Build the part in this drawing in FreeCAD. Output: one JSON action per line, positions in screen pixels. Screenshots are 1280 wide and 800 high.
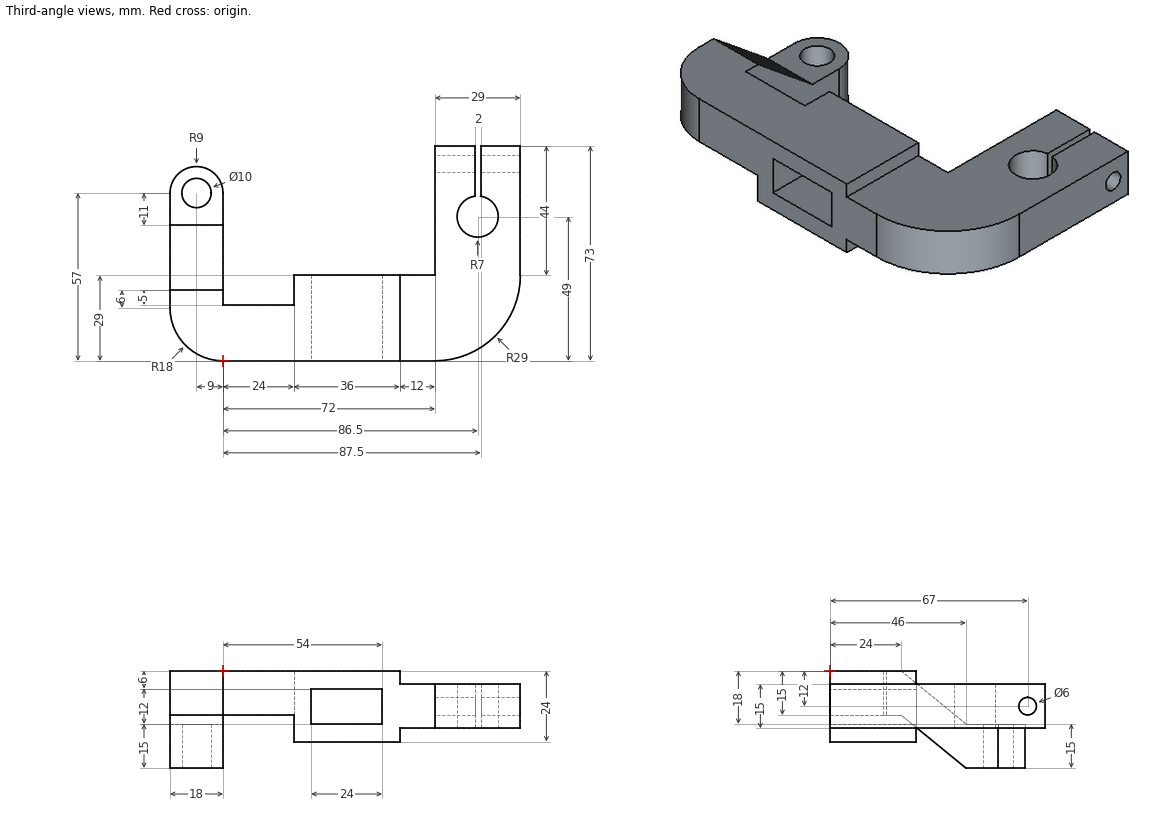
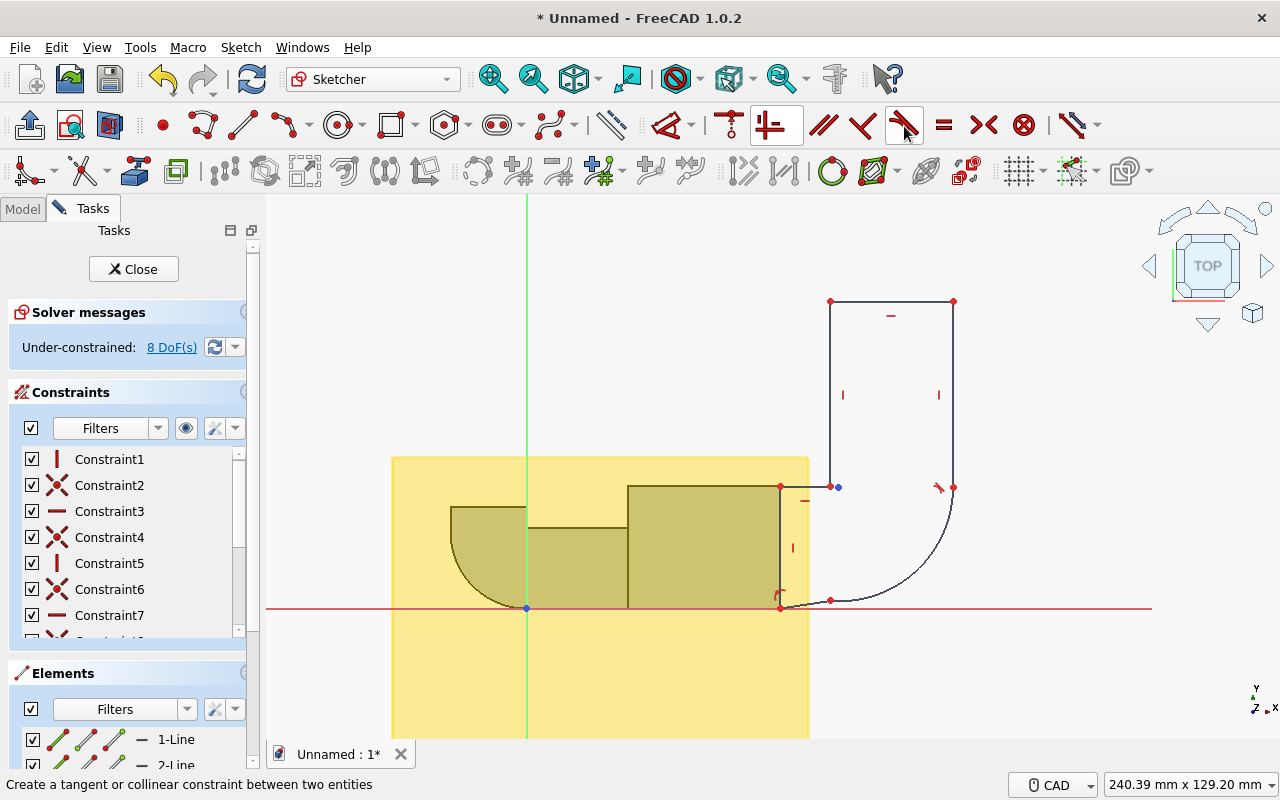
{"action": "left_click", "coordinate": [795, 606]}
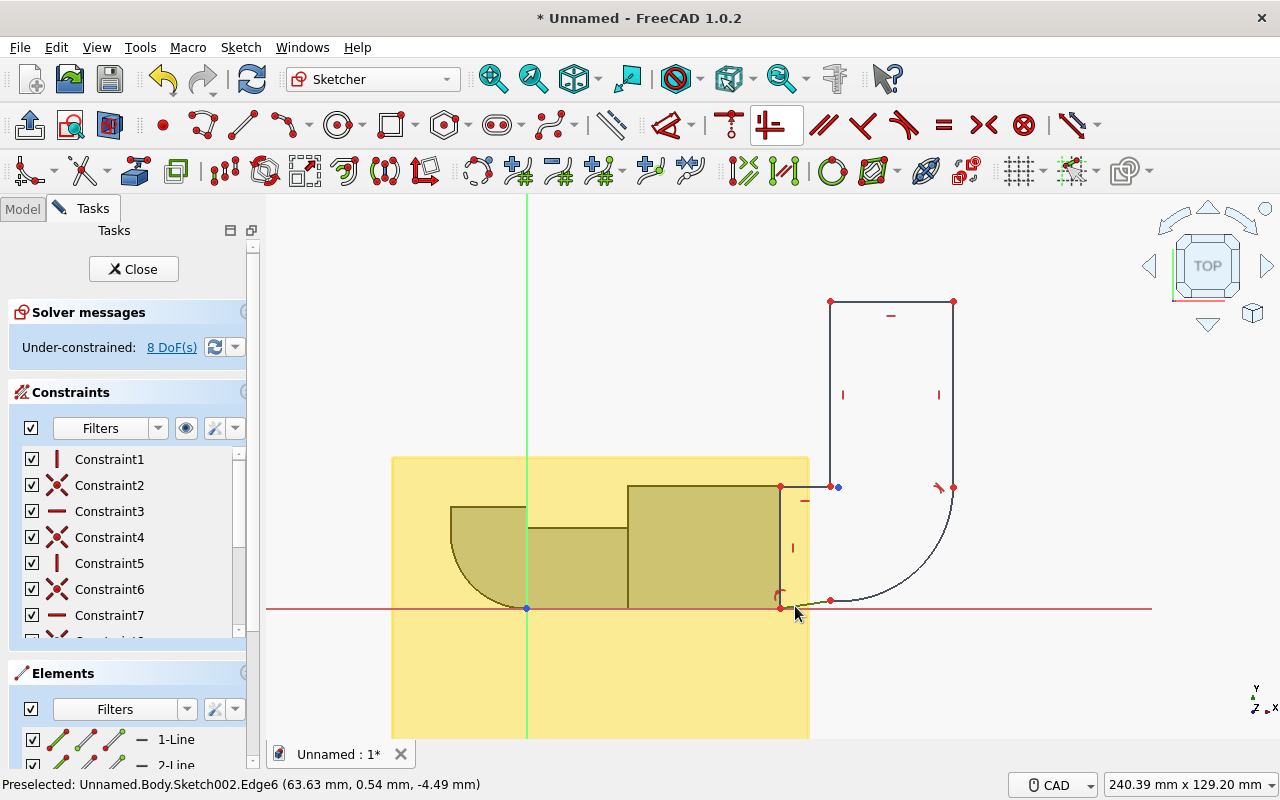
{"action": "left_click", "coordinate": [885, 591]}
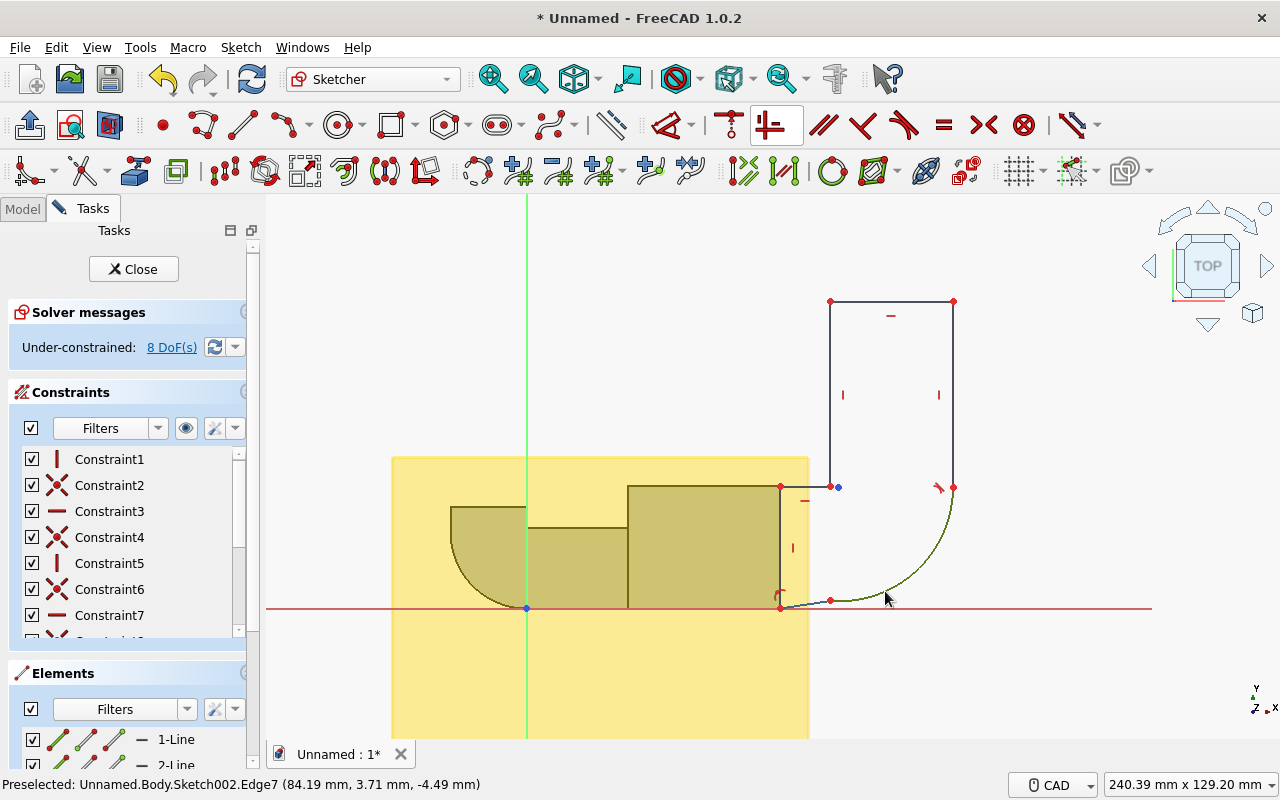
{"action": "left_click", "coordinate": [904, 126]}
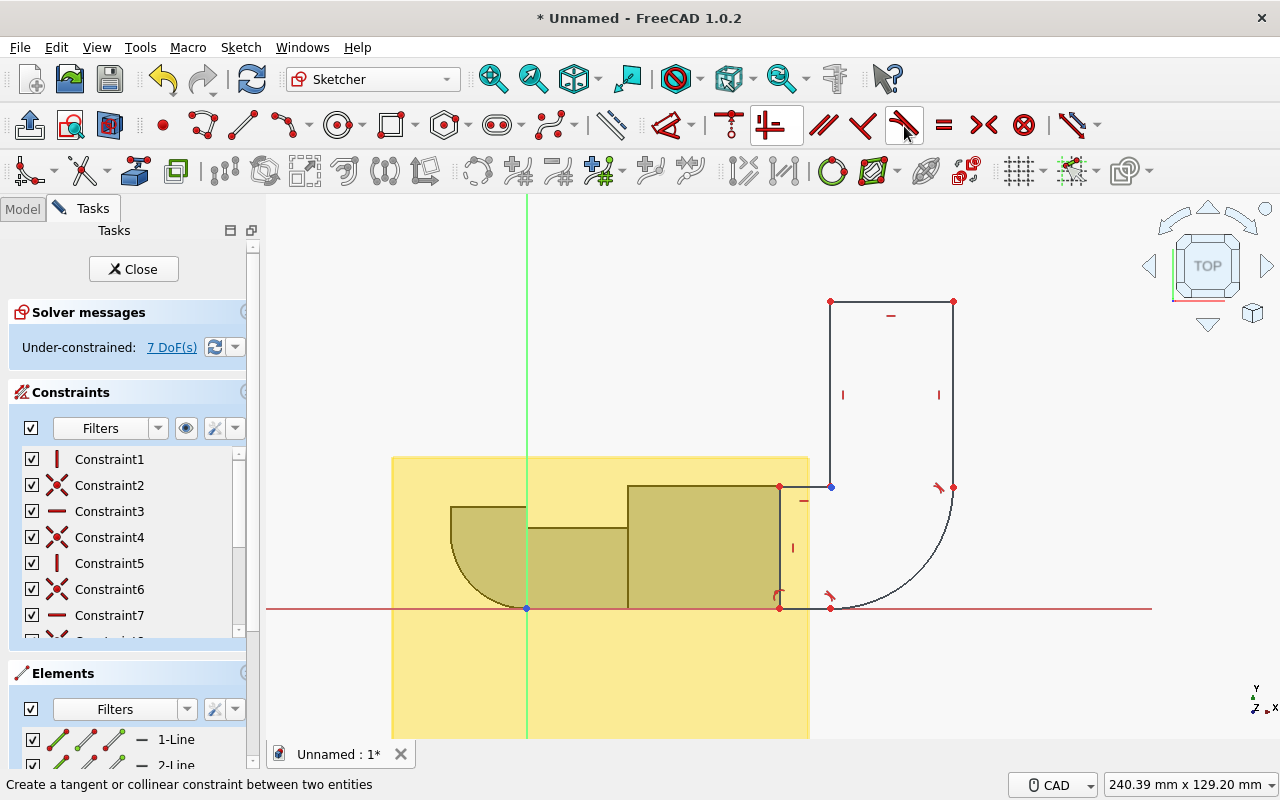
{"action": "left_click", "coordinate": [795, 609]}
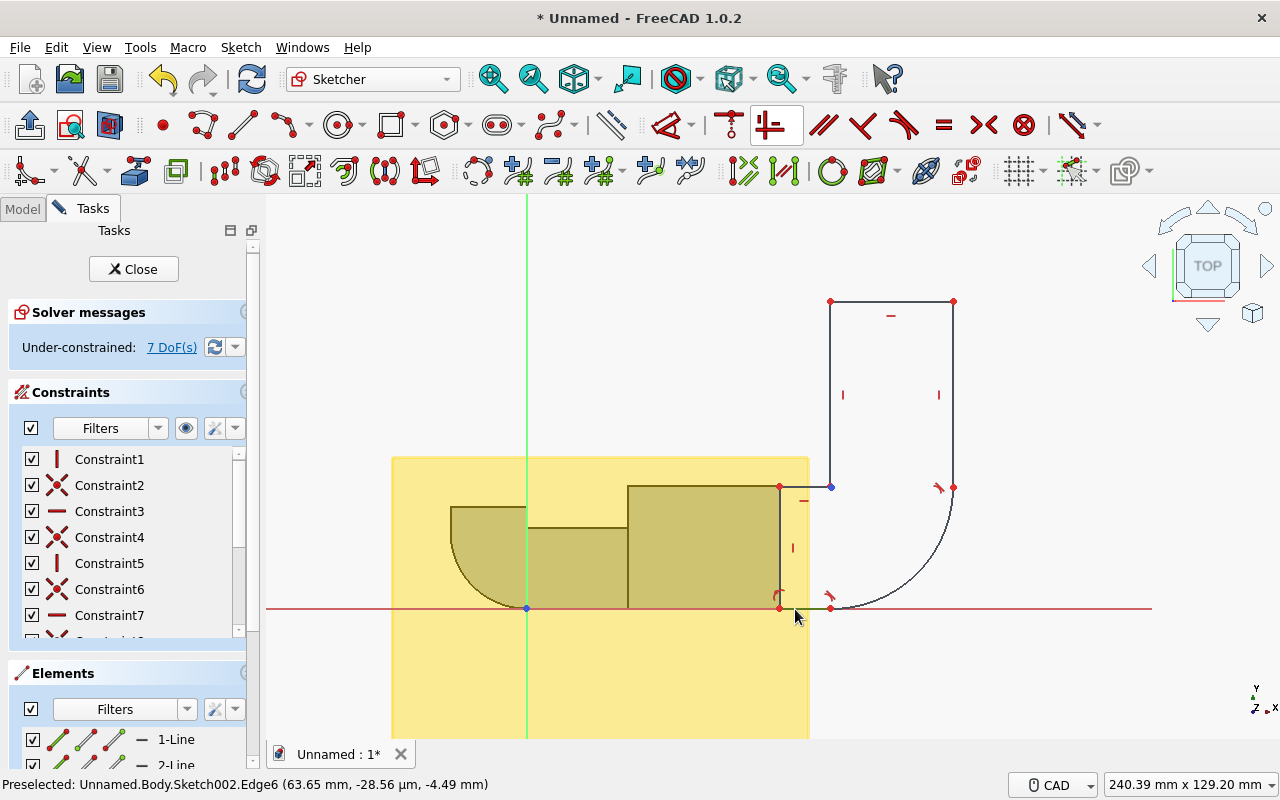
{"action": "left_click", "coordinate": [798, 126]}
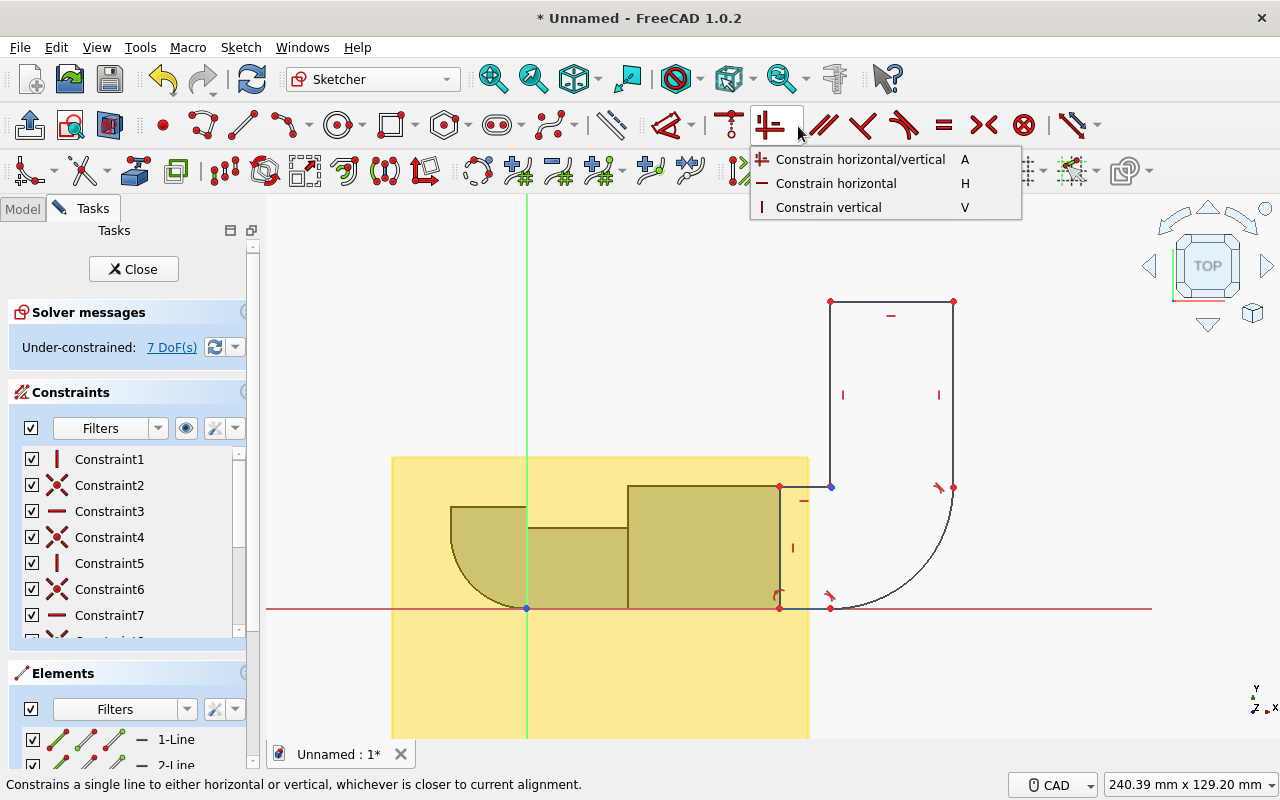
{"action": "left_click", "coordinate": [886, 183]}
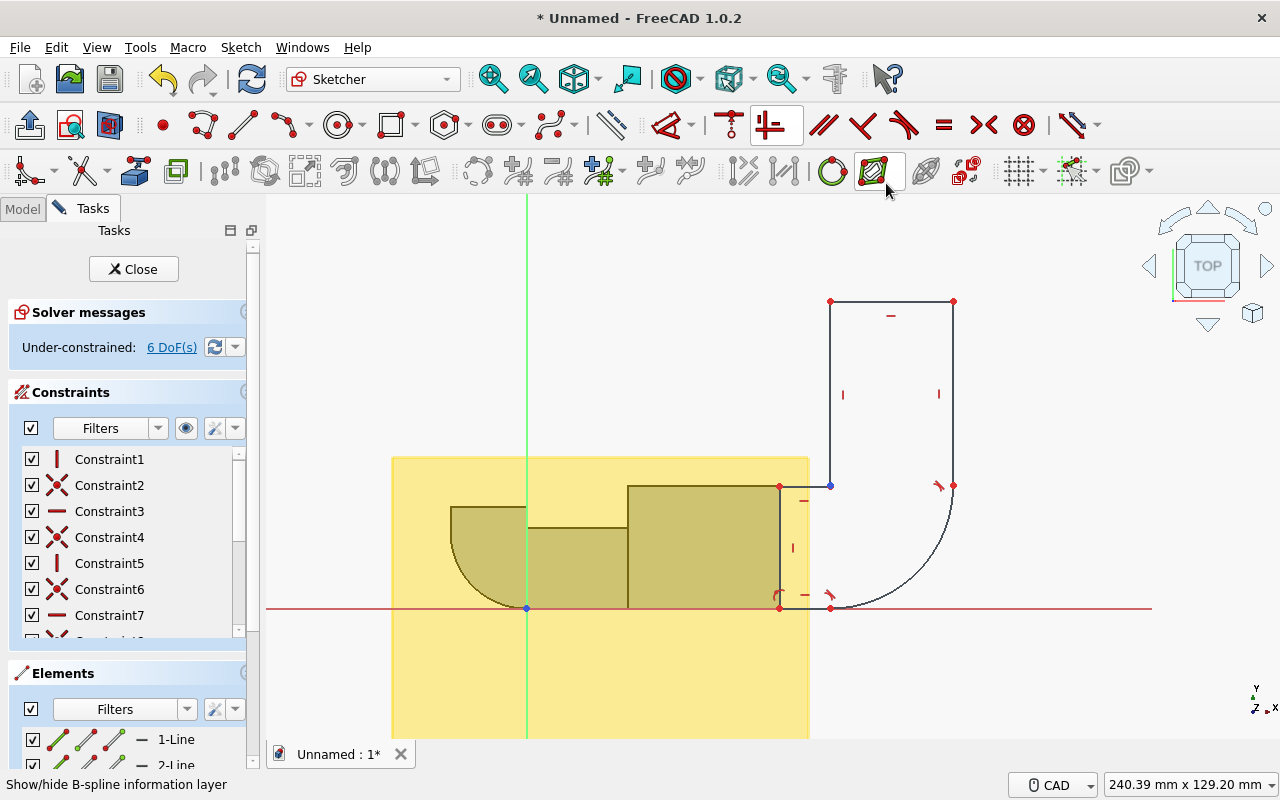
{"action": "left_click", "coordinate": [666, 126]}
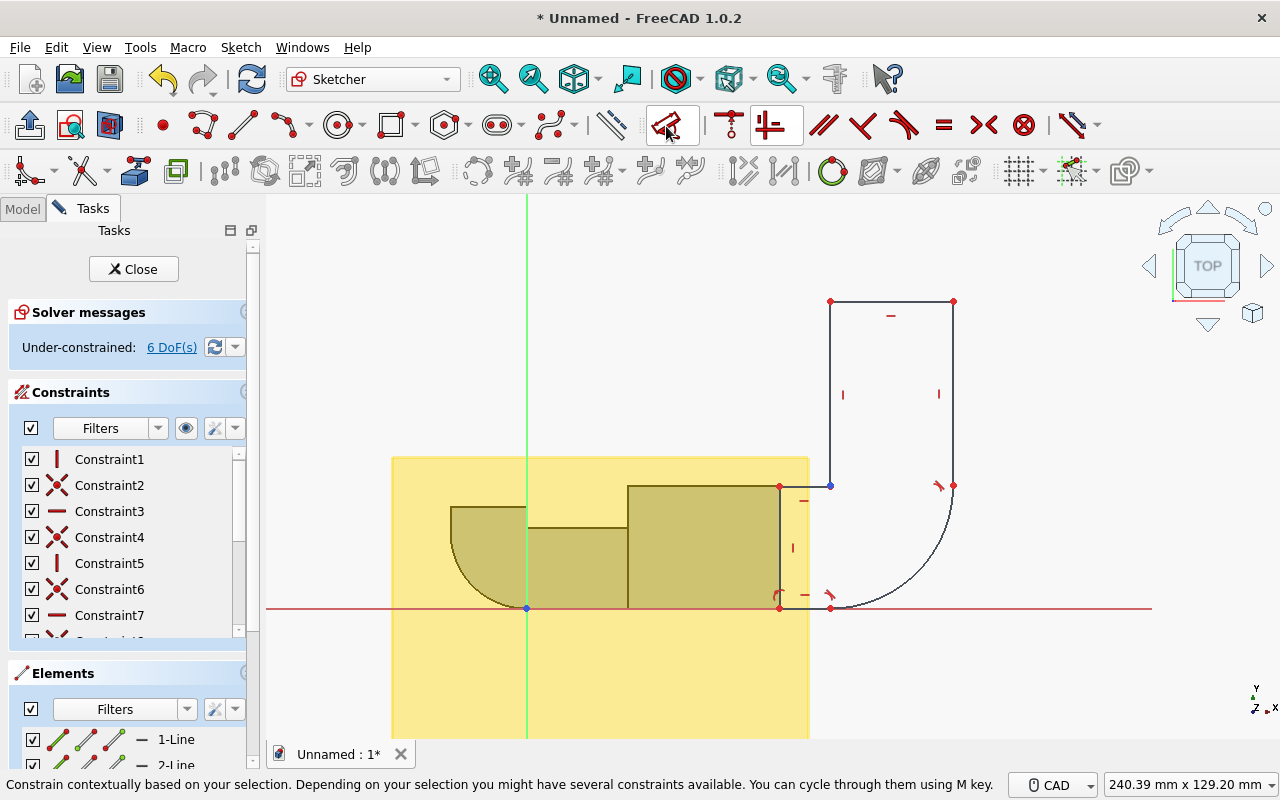
{"action": "left_click", "coordinate": [886, 595]}
{"action": "left_click", "coordinate": [901, 623]}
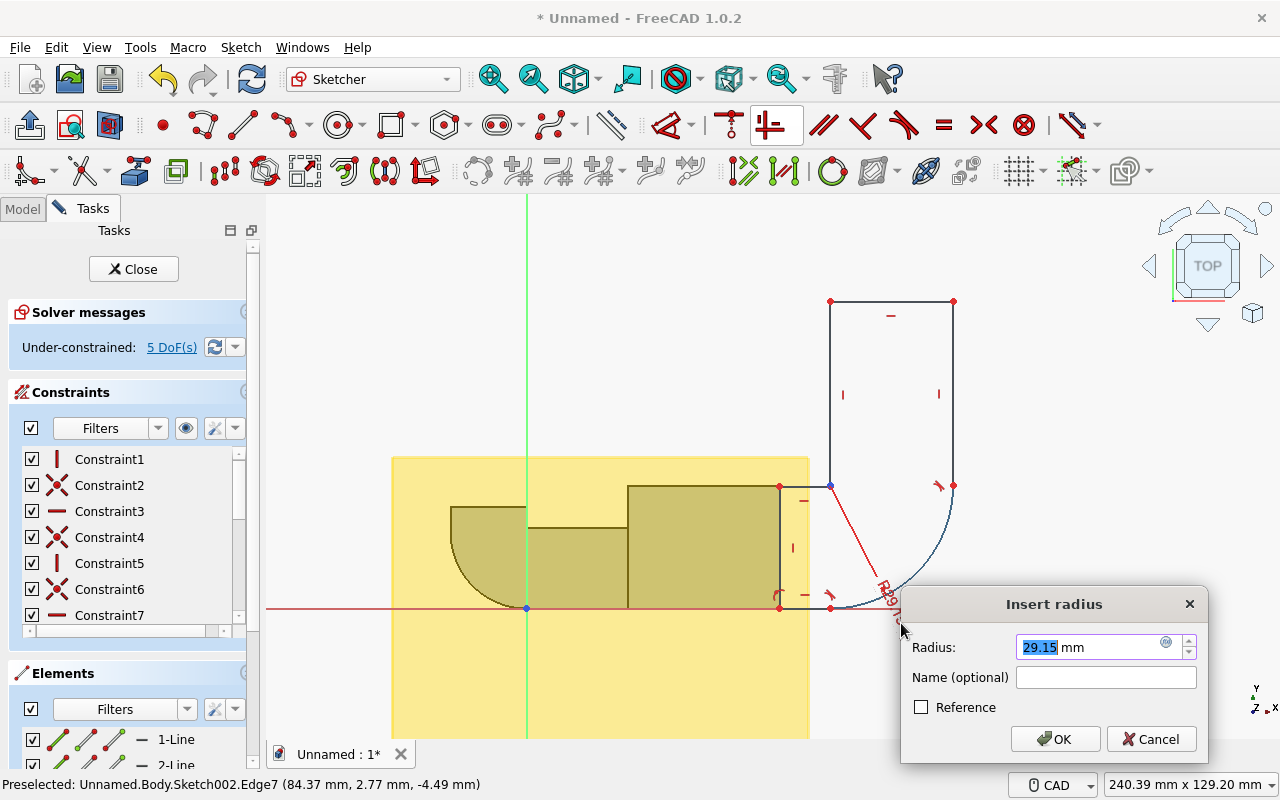
{"action": "type", "text": "29"}
{"action": "key", "text": "Return"}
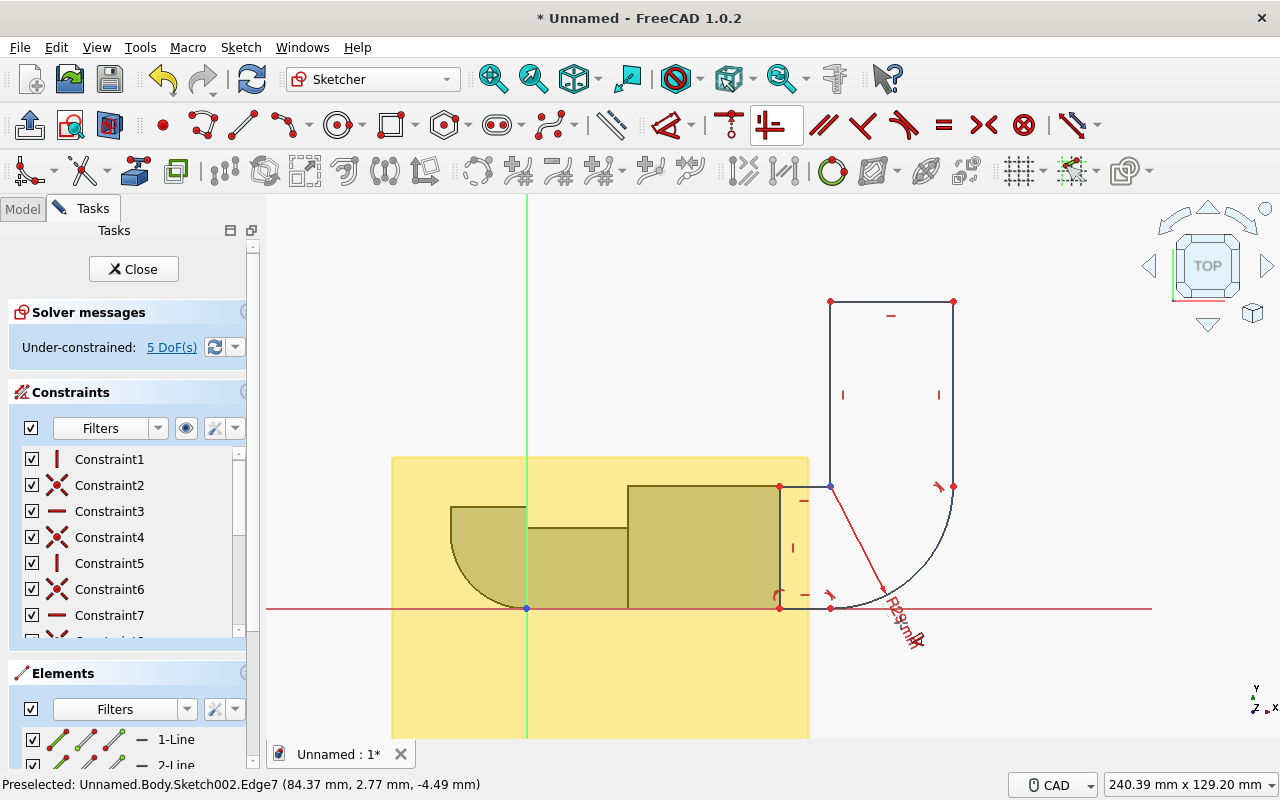
{"action": "left_click", "coordinate": [953, 431]}
{"action": "left_click", "coordinate": [987, 394]}